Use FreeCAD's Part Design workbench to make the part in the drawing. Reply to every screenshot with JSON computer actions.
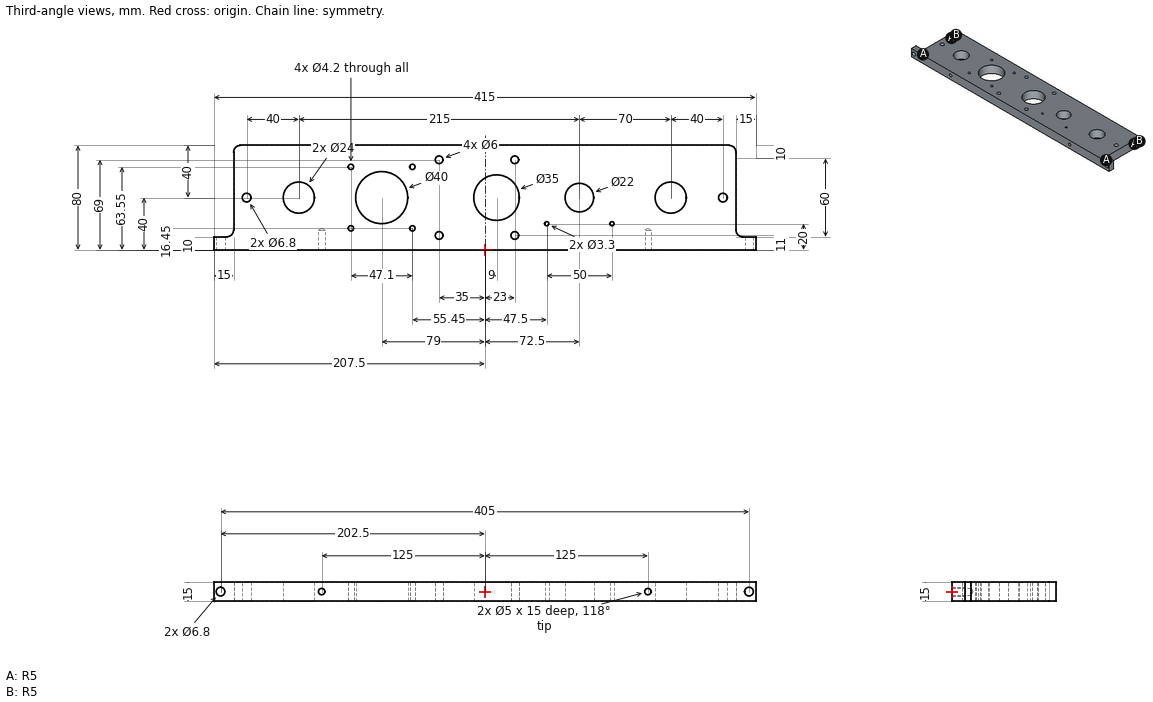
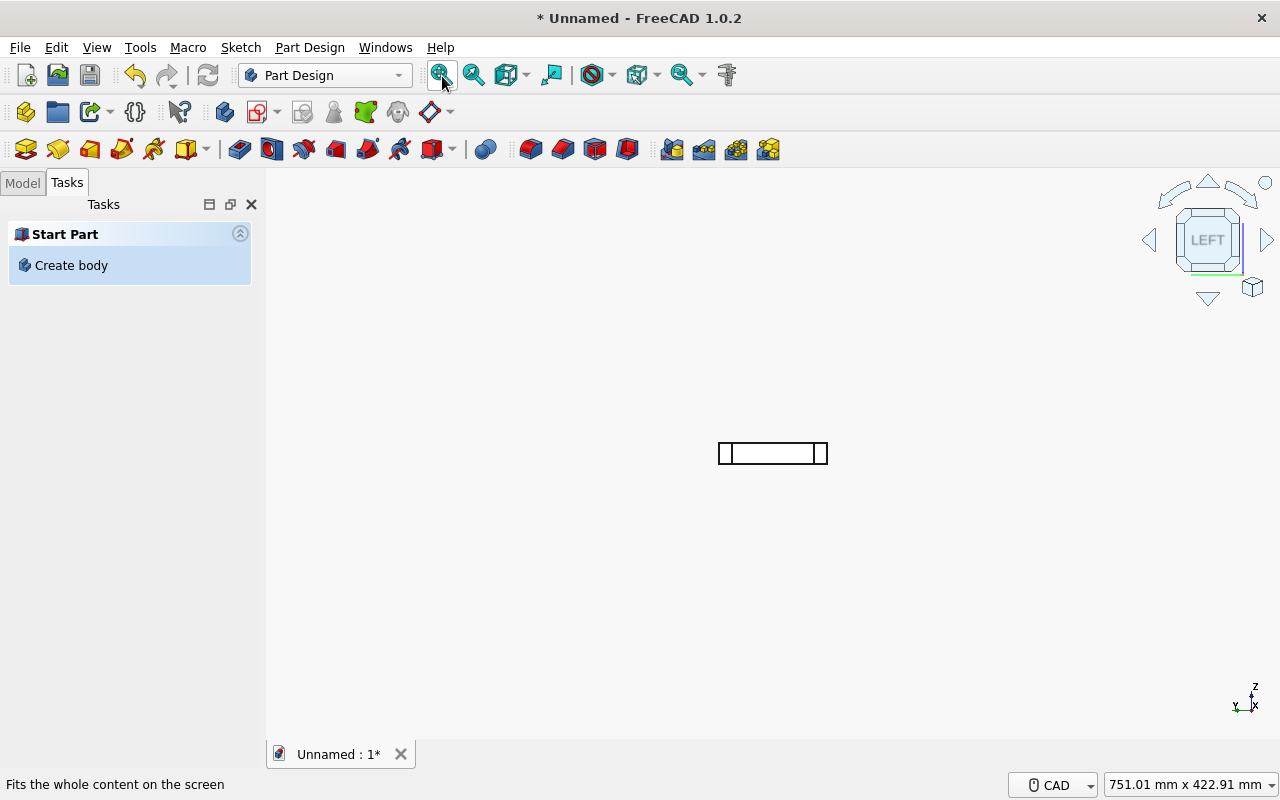
{"action": "left_click", "coordinate": [442, 76]}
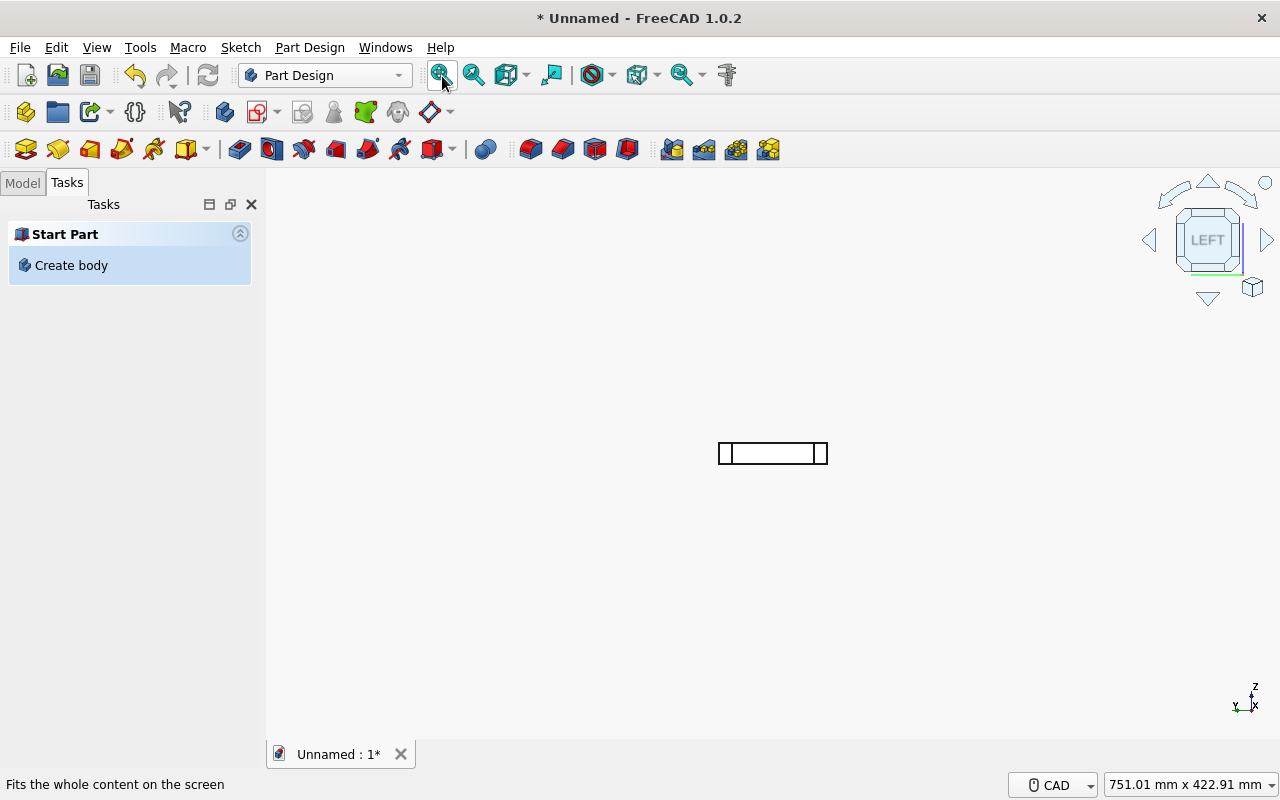
{"action": "scroll", "coordinate": [814, 452], "scroll_direction": "up", "scroll_amount": 4}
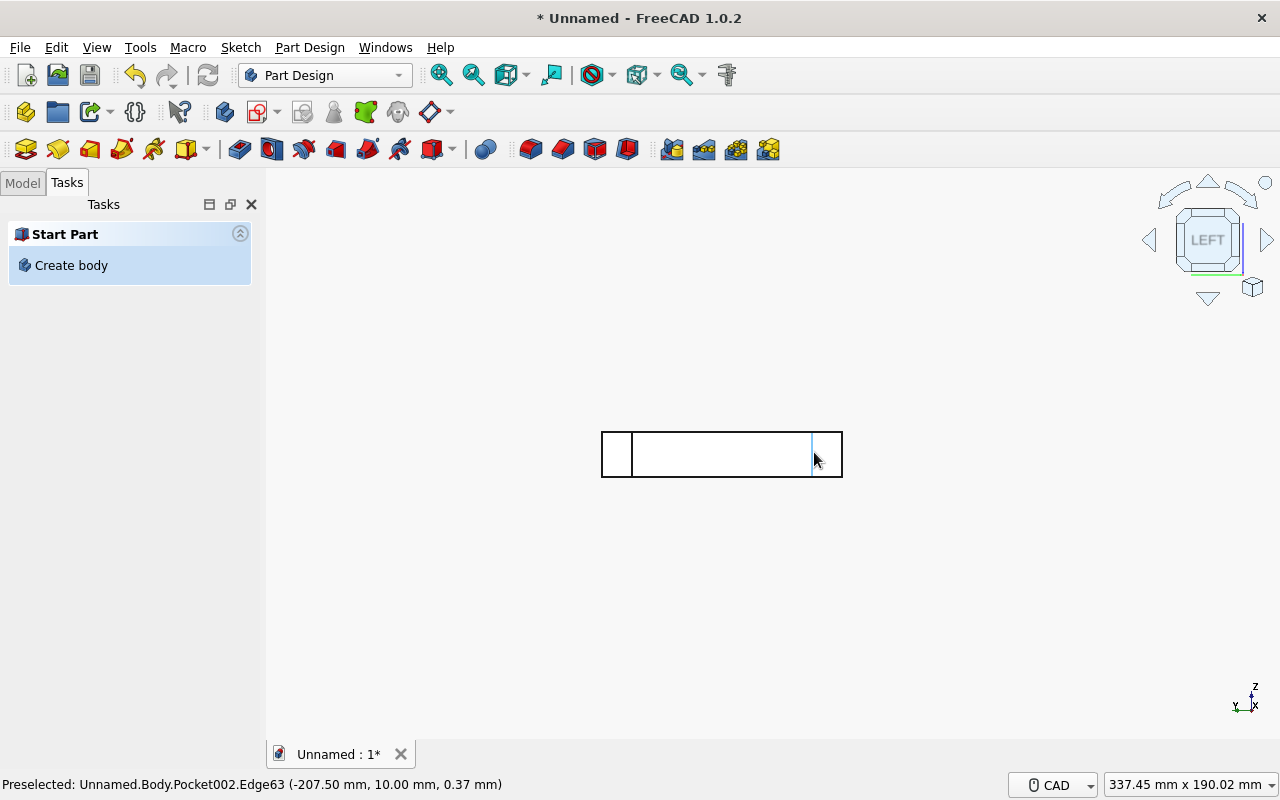
{"action": "left_click", "coordinate": [442, 76]}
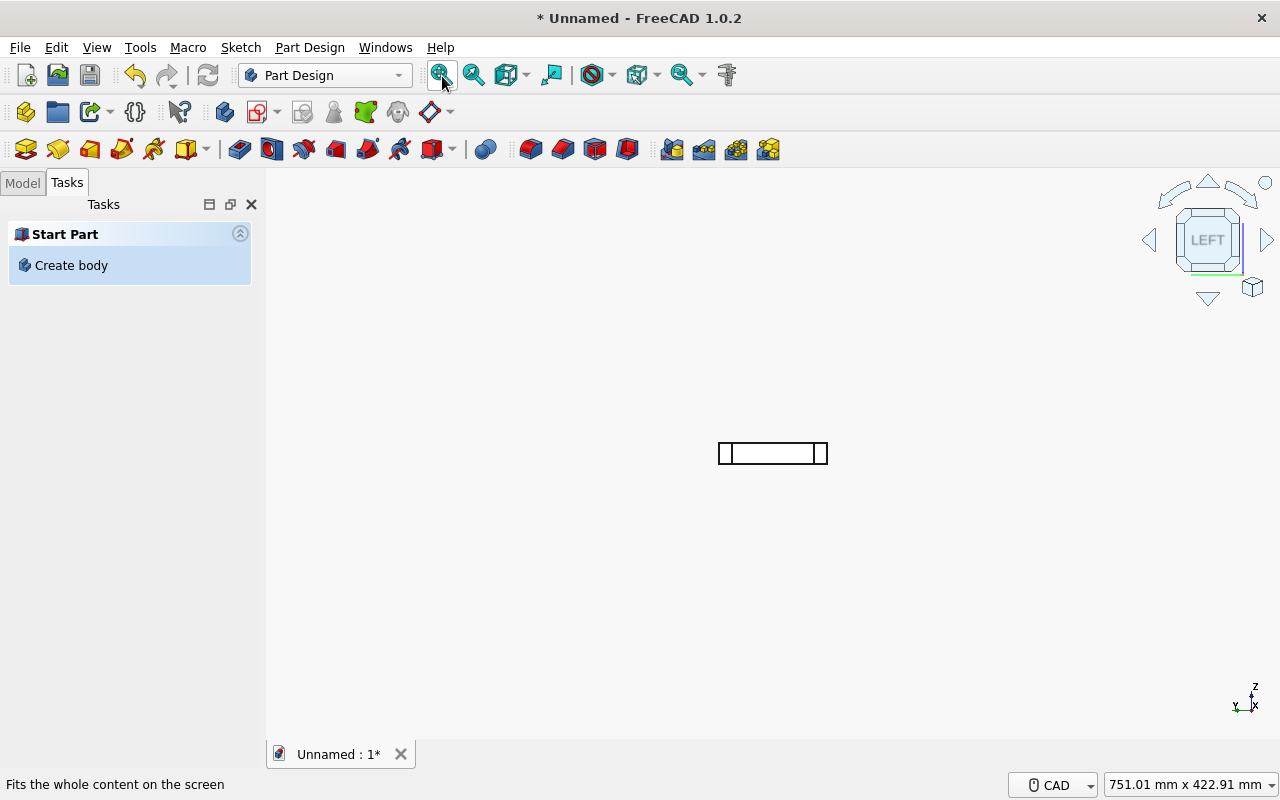
{"action": "key", "text": "v 3"}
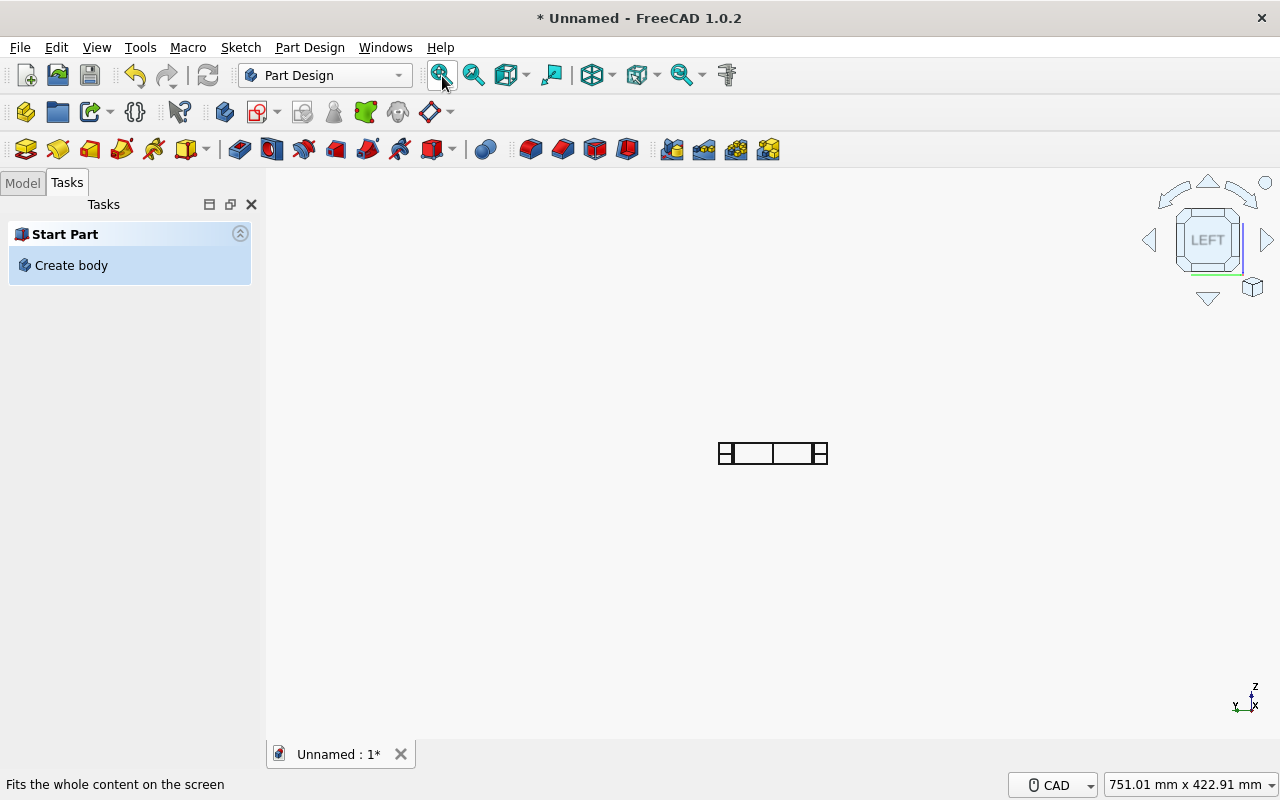
{"action": "key", "text": "0"}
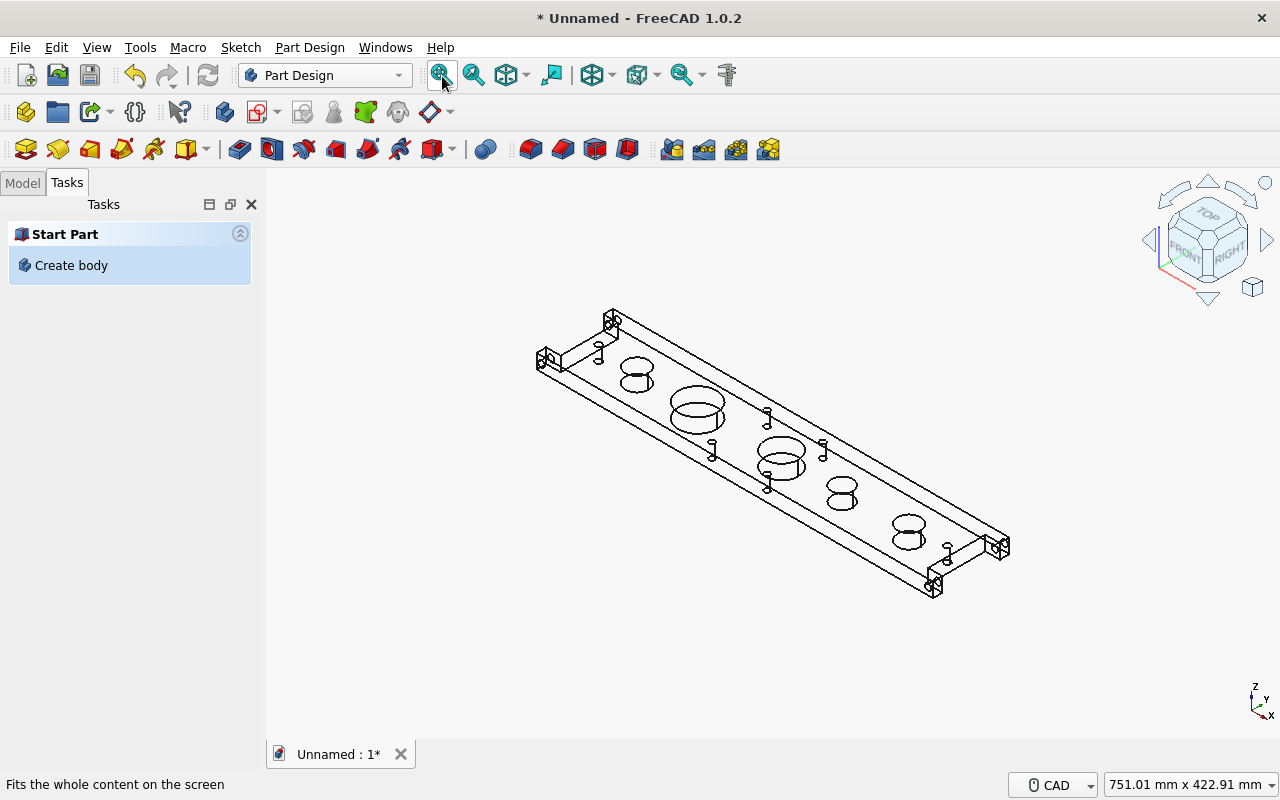
{"action": "left_click", "coordinate": [618, 330]}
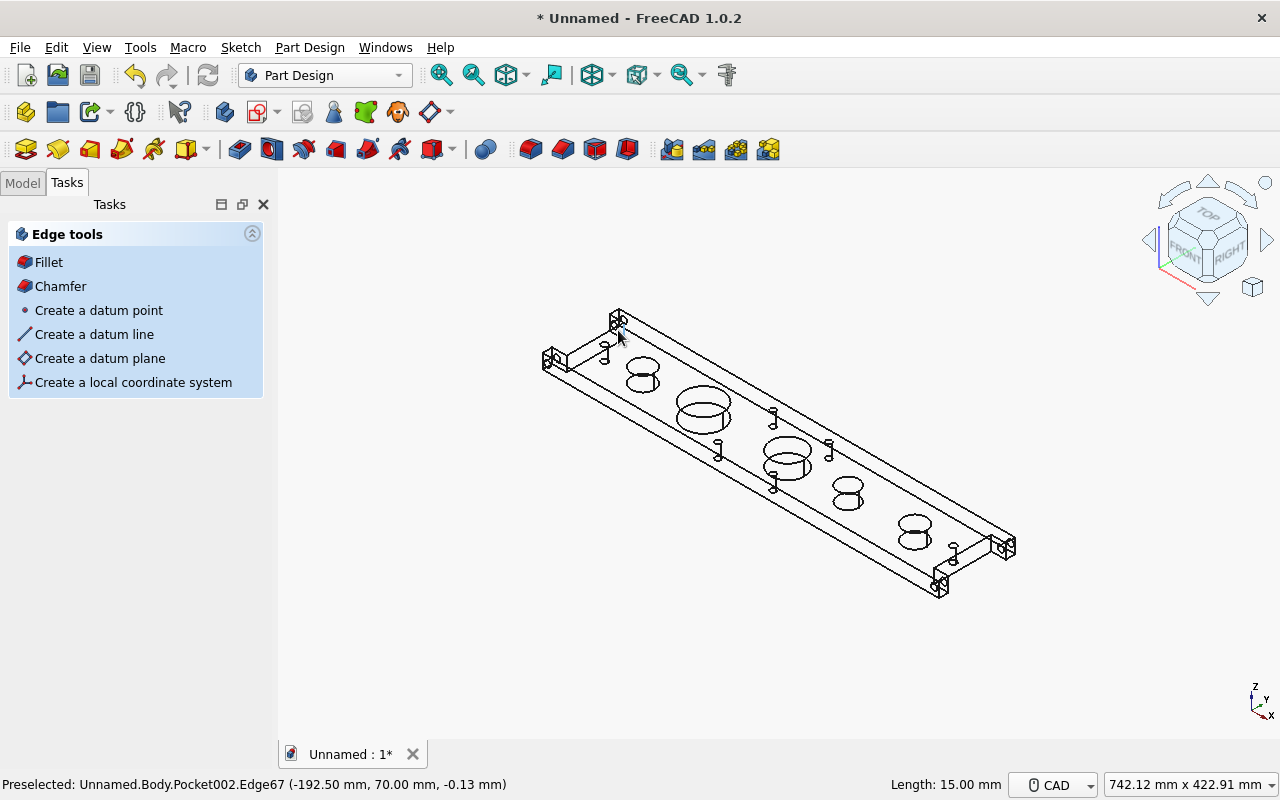
{"action": "left_click", "coordinate": [991, 542], "text": "ctrl"}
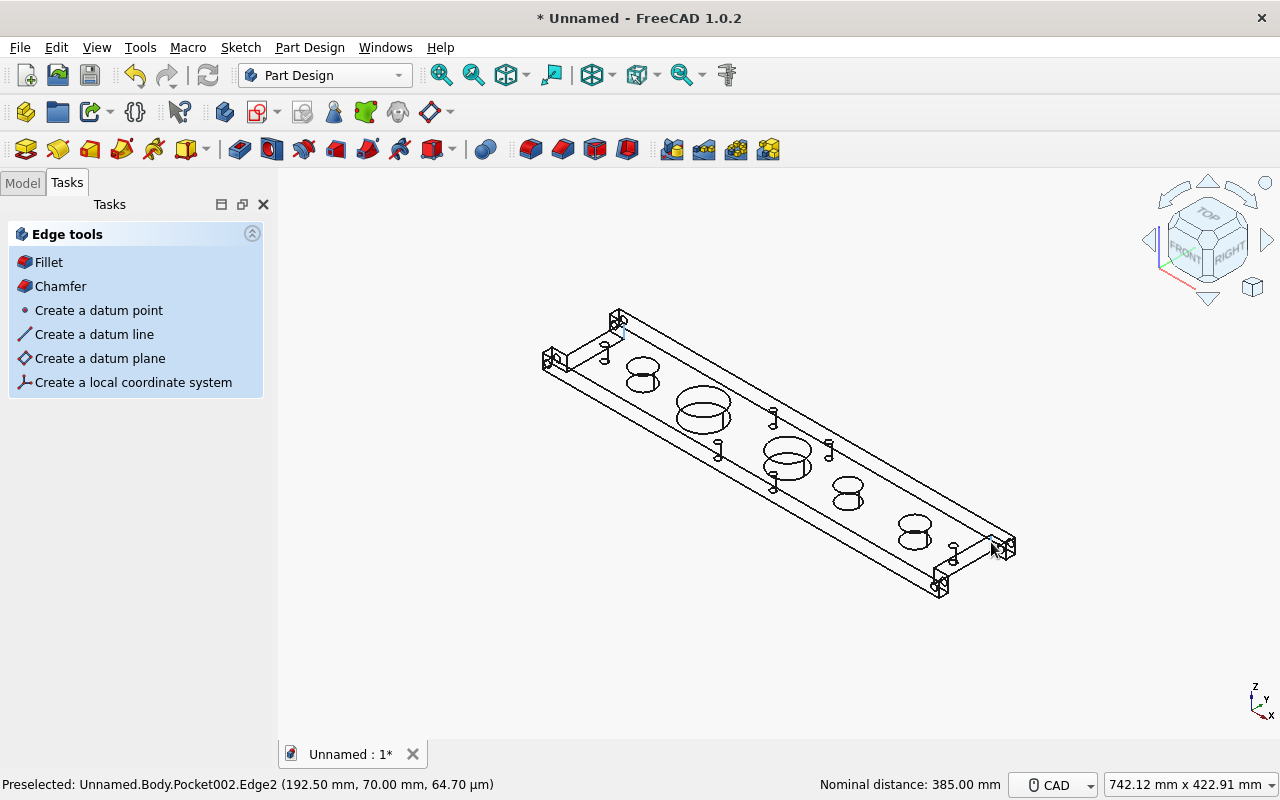
{"action": "scroll", "coordinate": [567, 363], "scroll_direction": "up", "scroll_amount": 6}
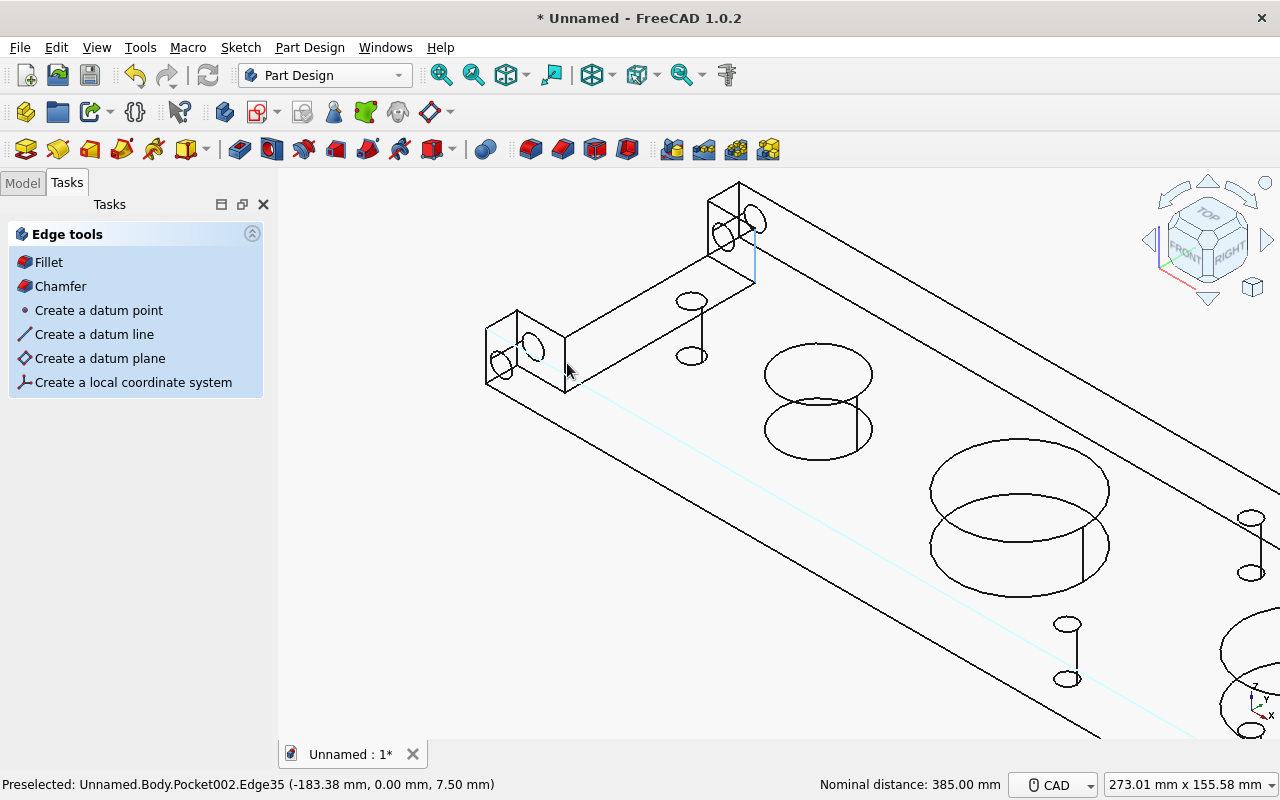
{"action": "left_click", "coordinate": [565, 364], "text": "ctrl"}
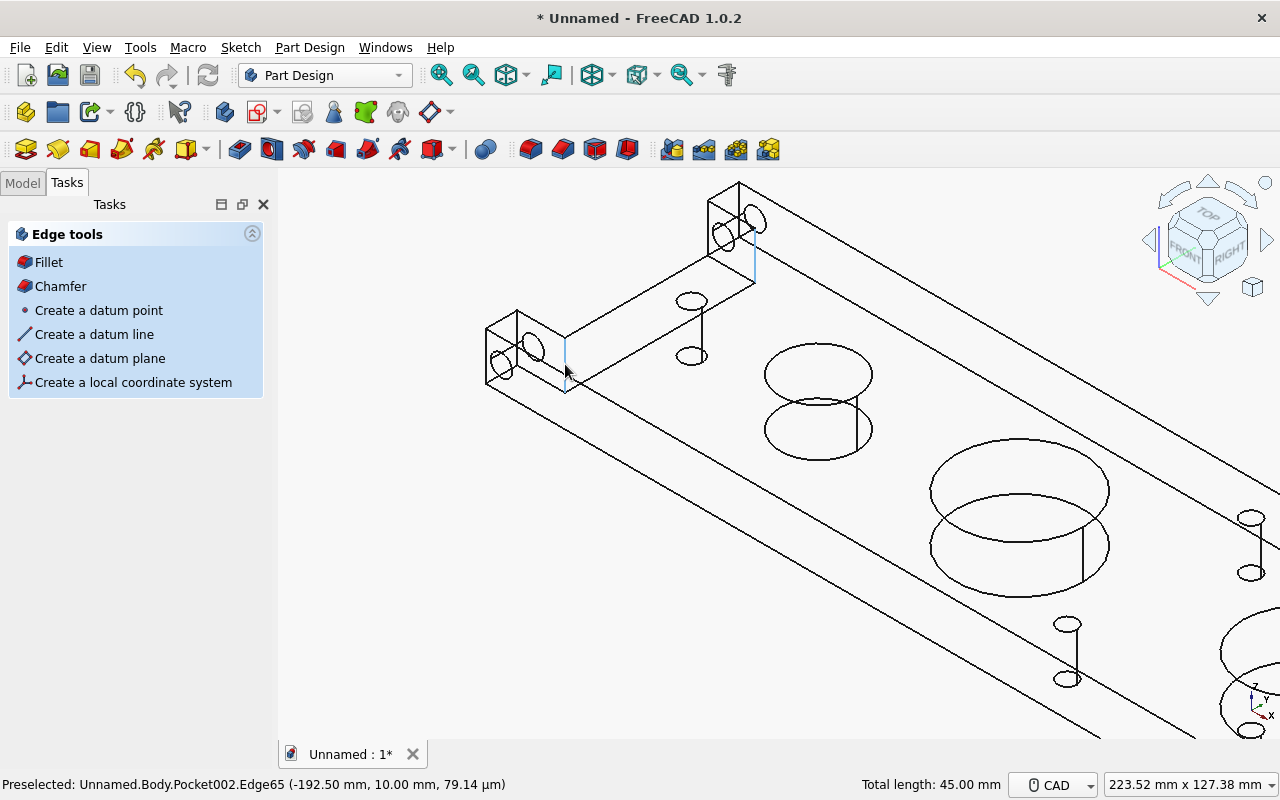
{"action": "left_click", "coordinate": [442, 76]}